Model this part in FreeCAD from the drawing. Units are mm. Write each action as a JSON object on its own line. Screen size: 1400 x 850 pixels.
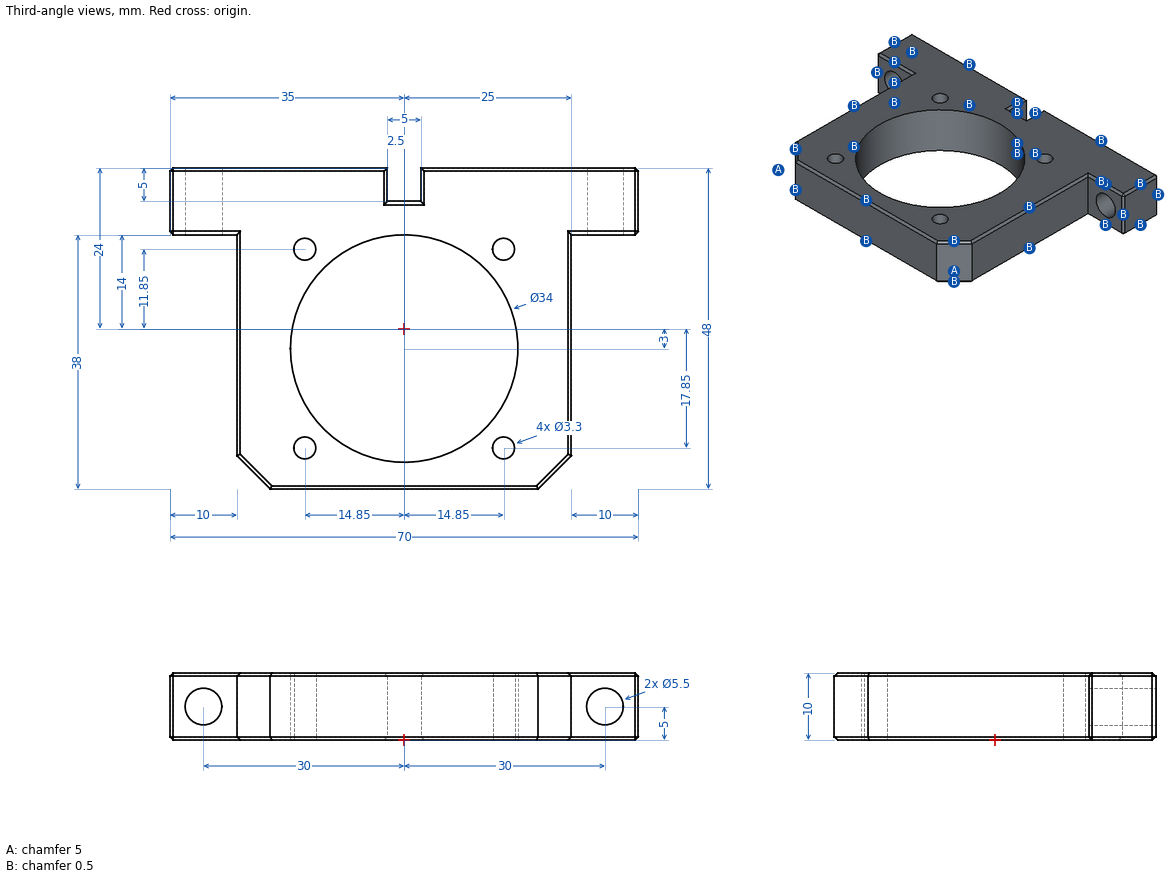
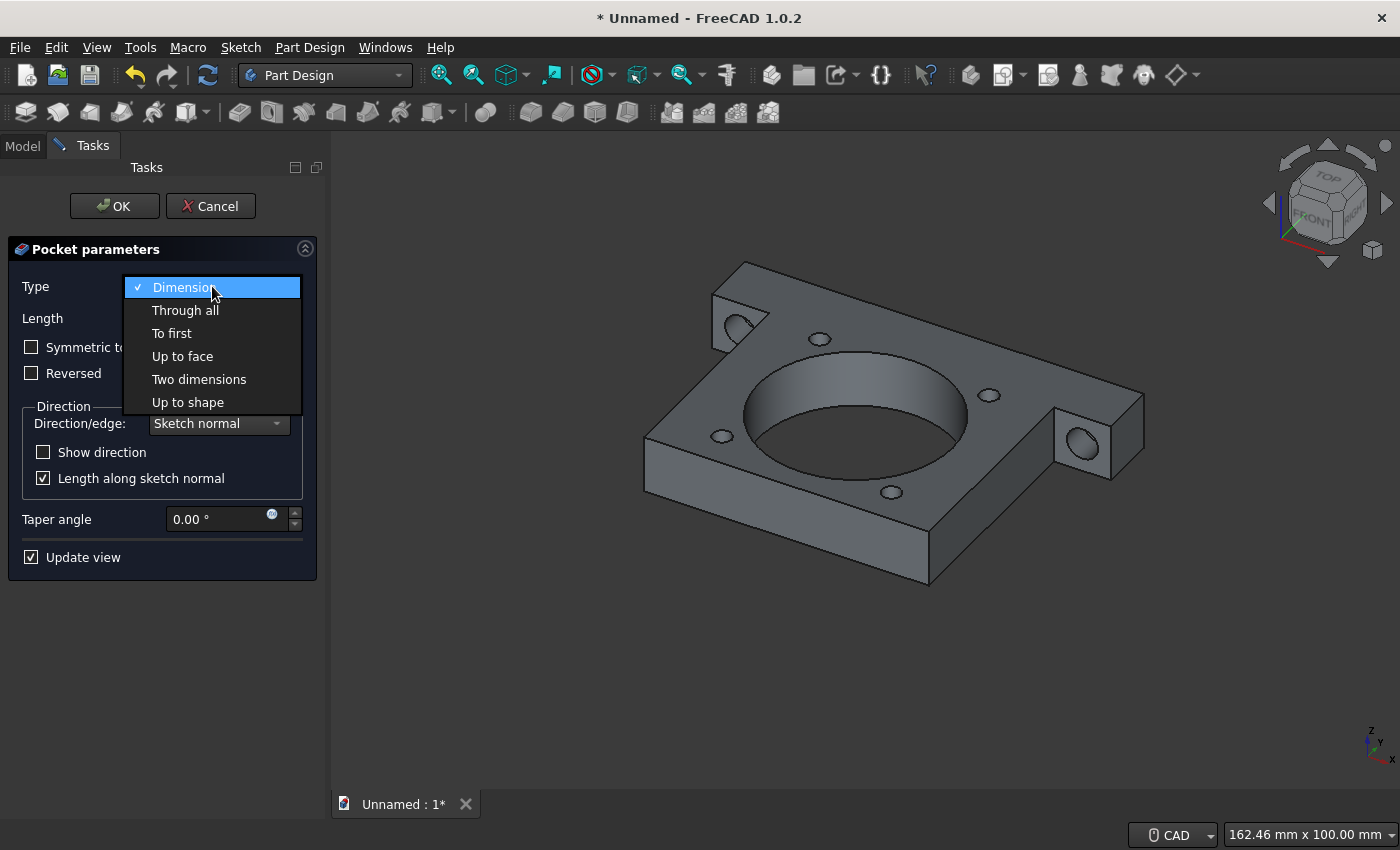
{"action": "left_click", "coordinate": [212, 310]}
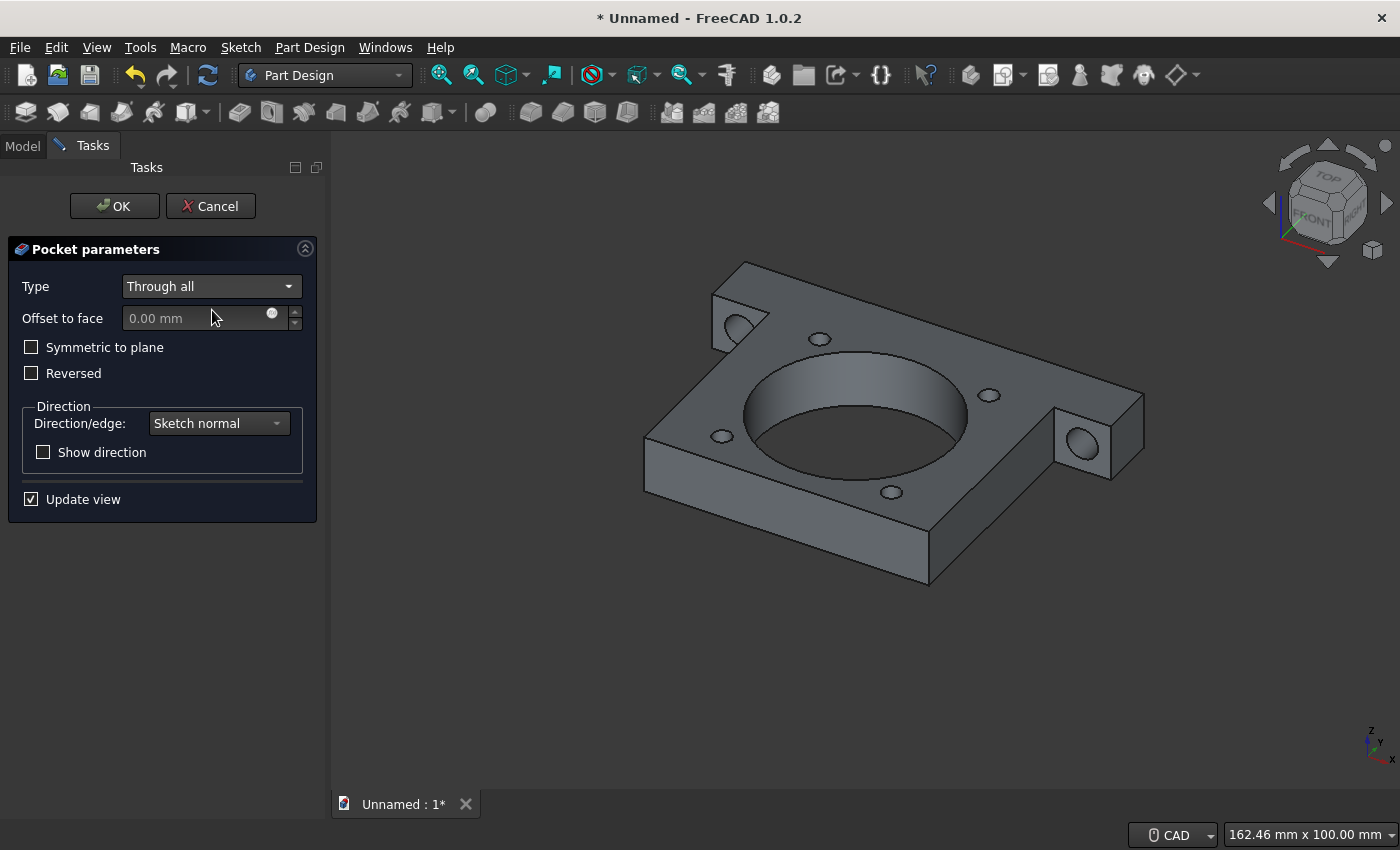
{"action": "left_click", "coordinate": [115, 206]}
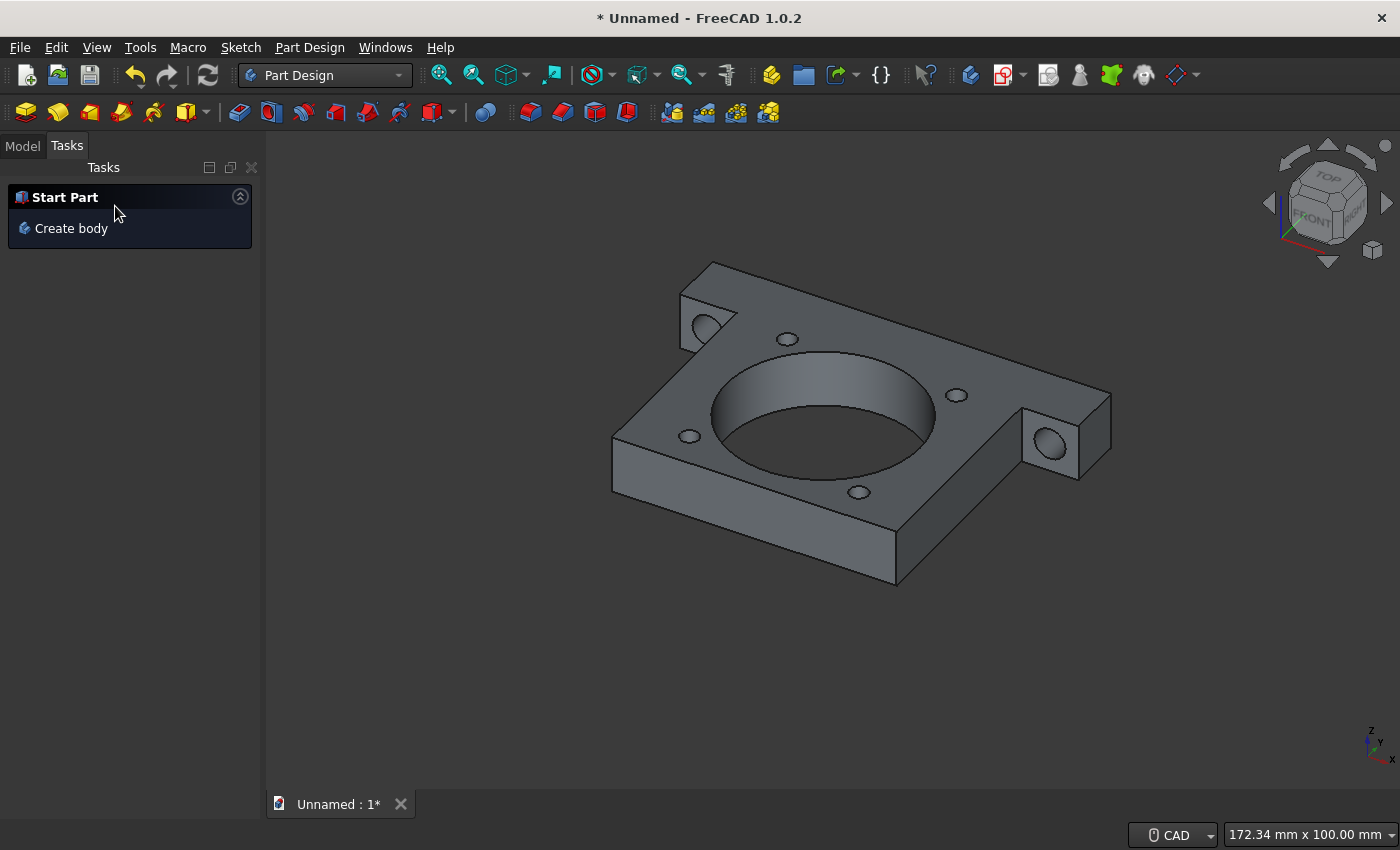
{"action": "left_click", "coordinate": [897, 558]}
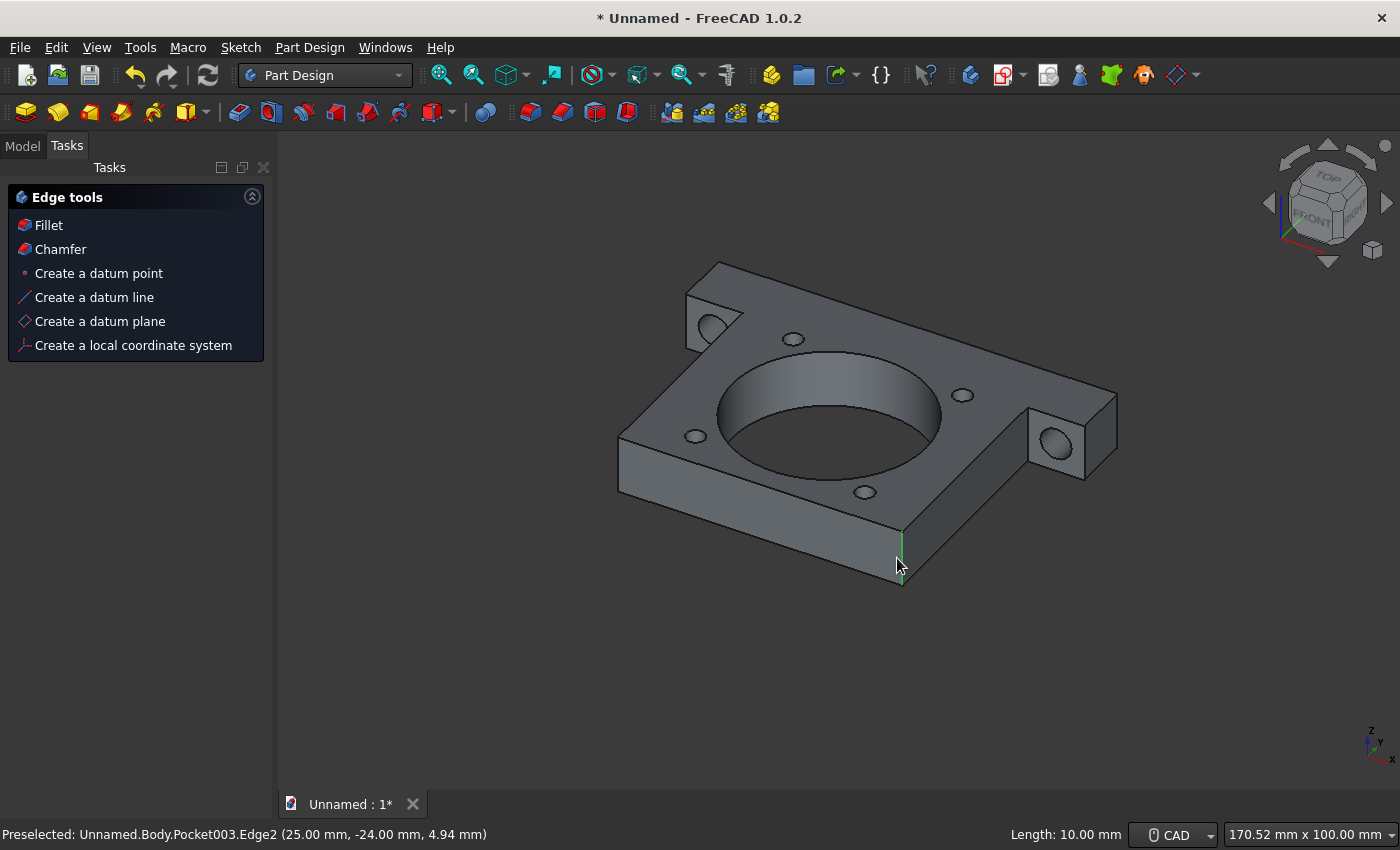
{"action": "key", "text": "0"}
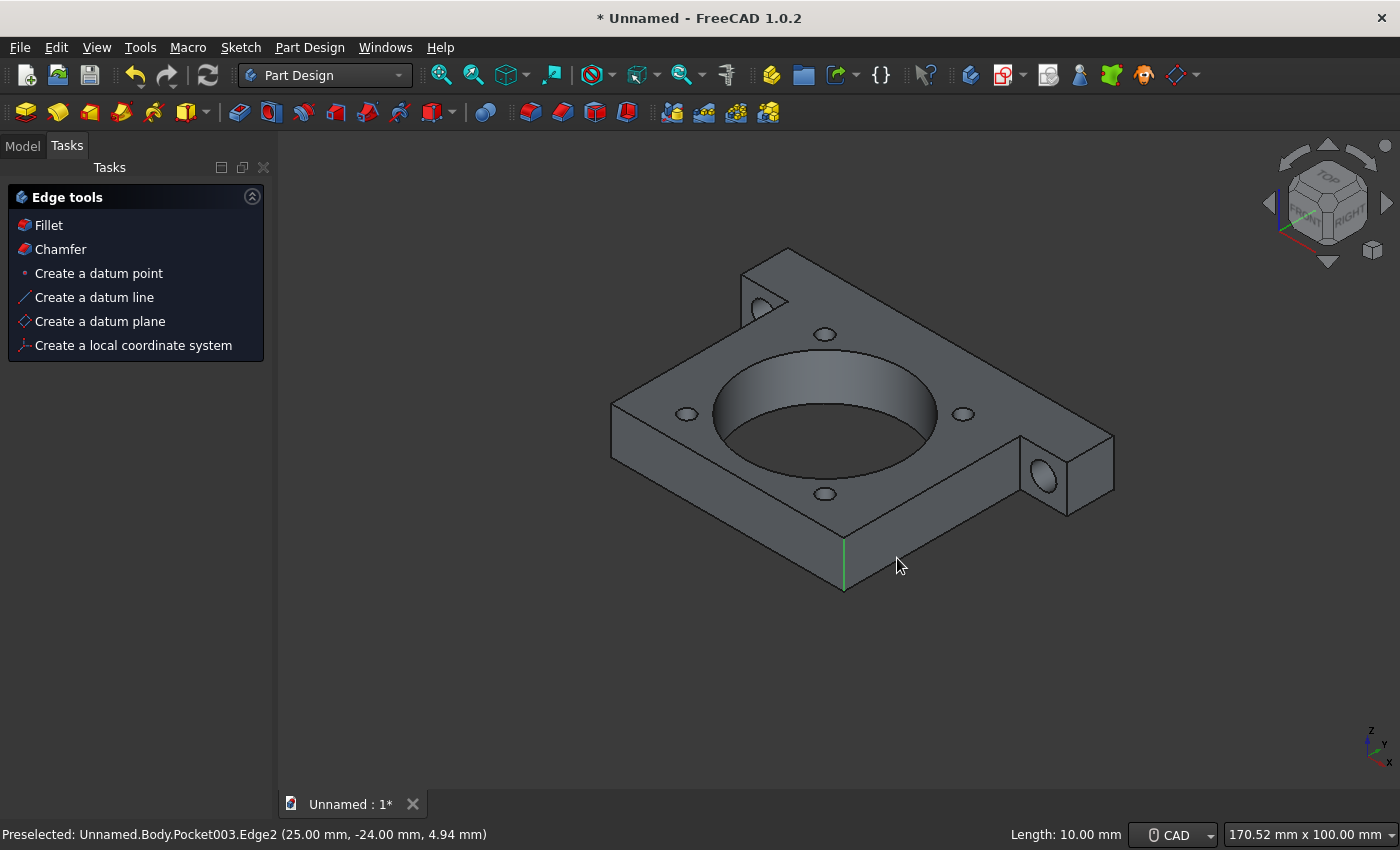
{"action": "key", "text": "2"}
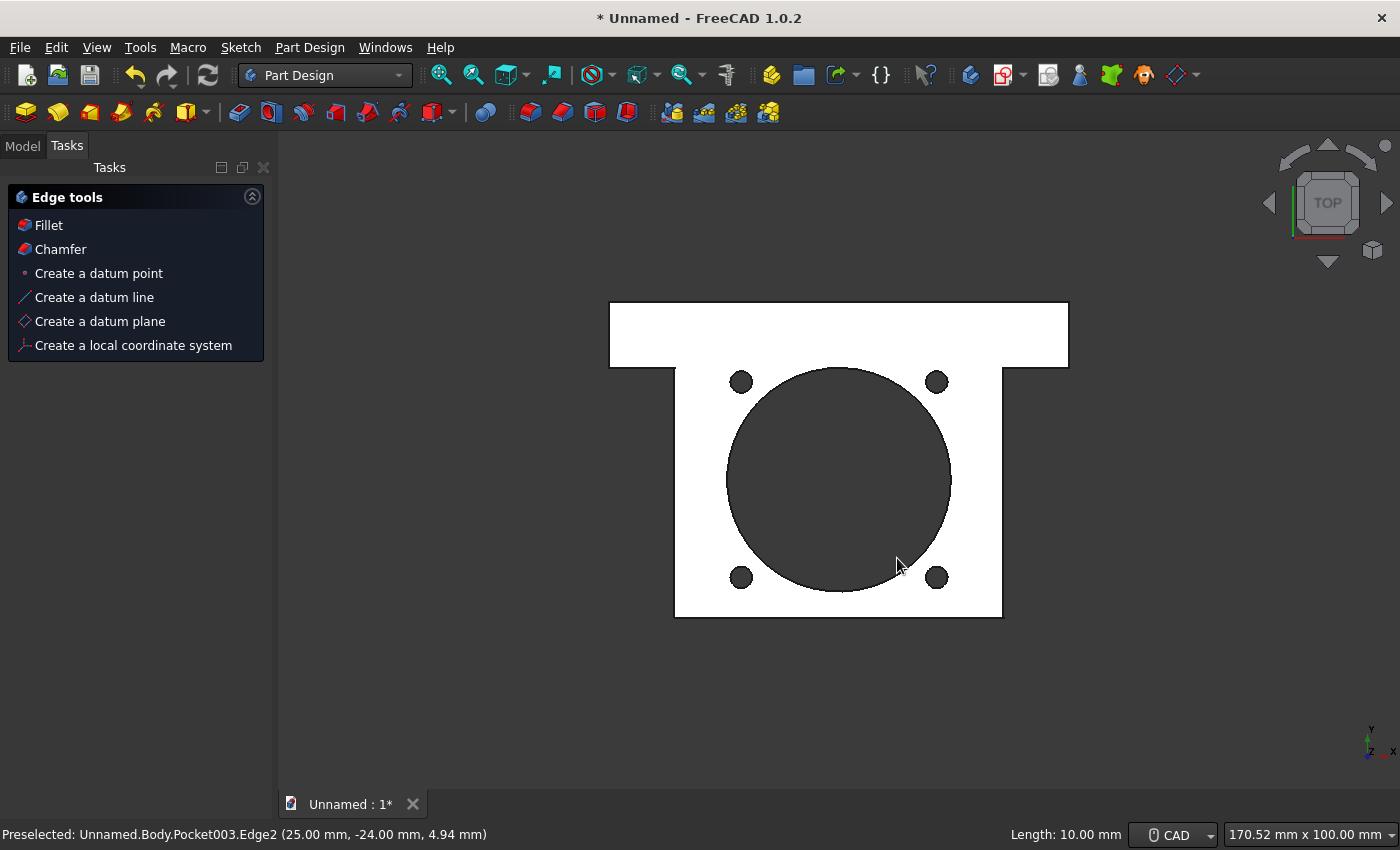
{"action": "key", "text": "1"}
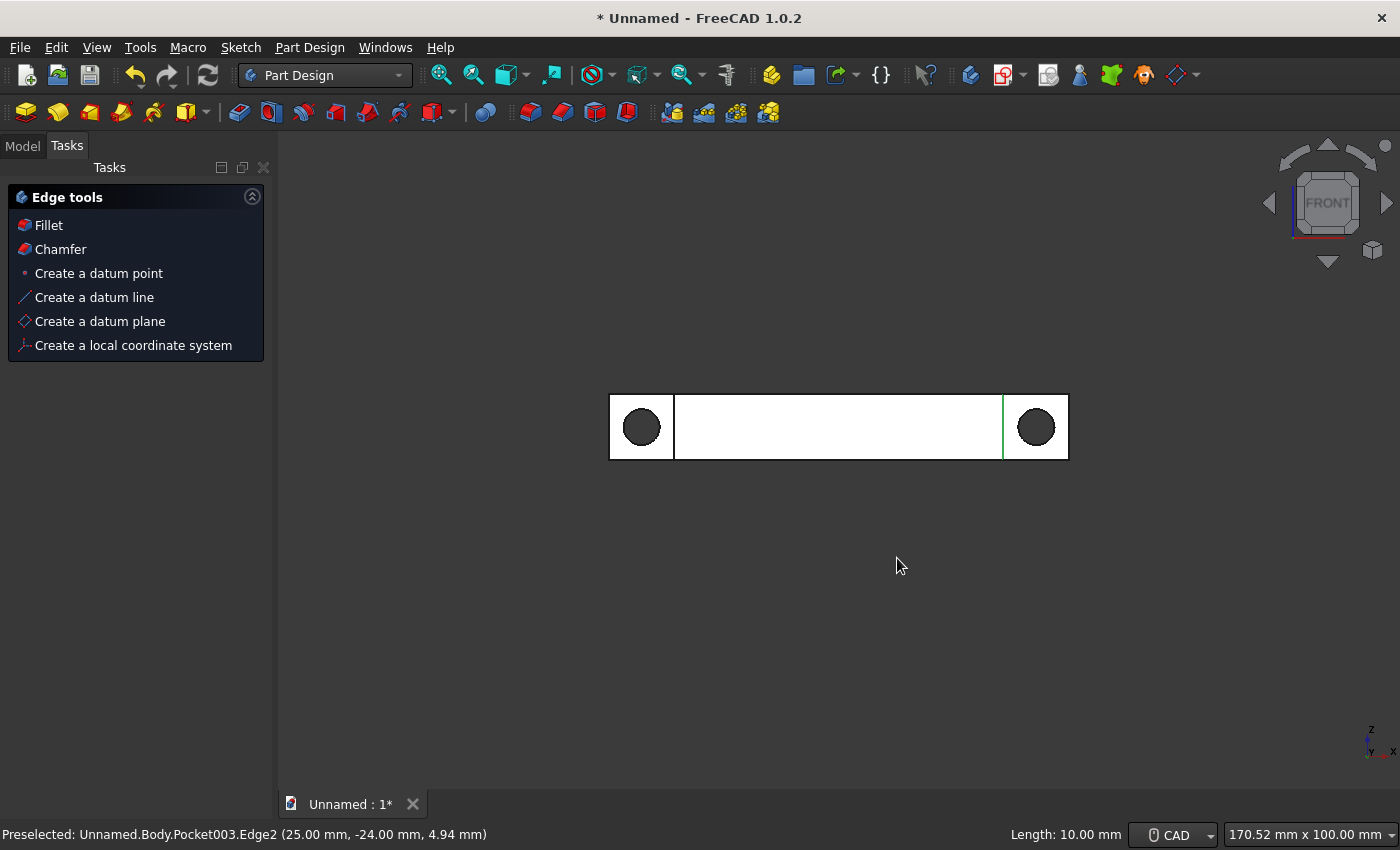
{"action": "left_click", "coordinate": [442, 76]}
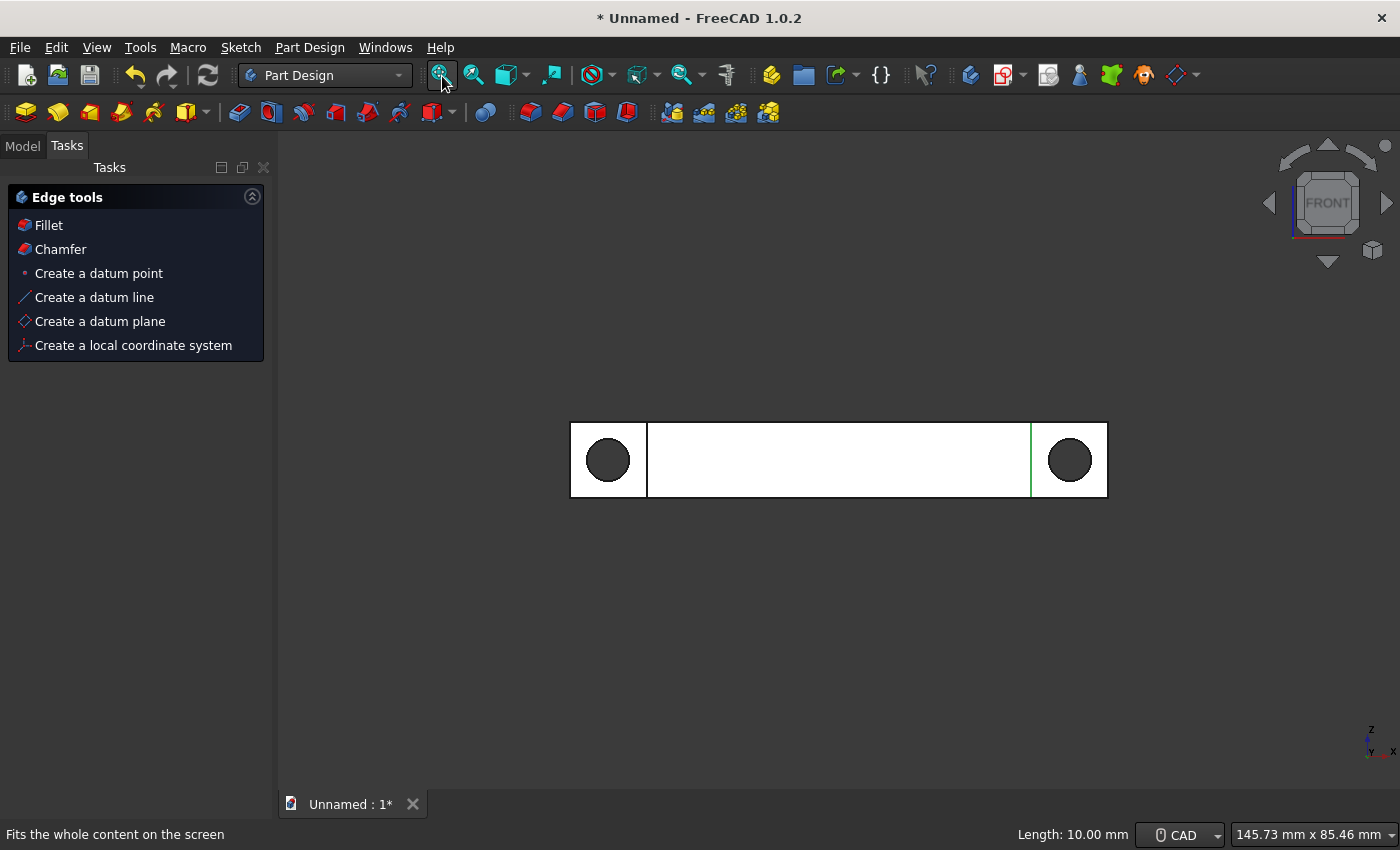
{"action": "left_click", "coordinate": [647, 459], "text": "ctrl"}